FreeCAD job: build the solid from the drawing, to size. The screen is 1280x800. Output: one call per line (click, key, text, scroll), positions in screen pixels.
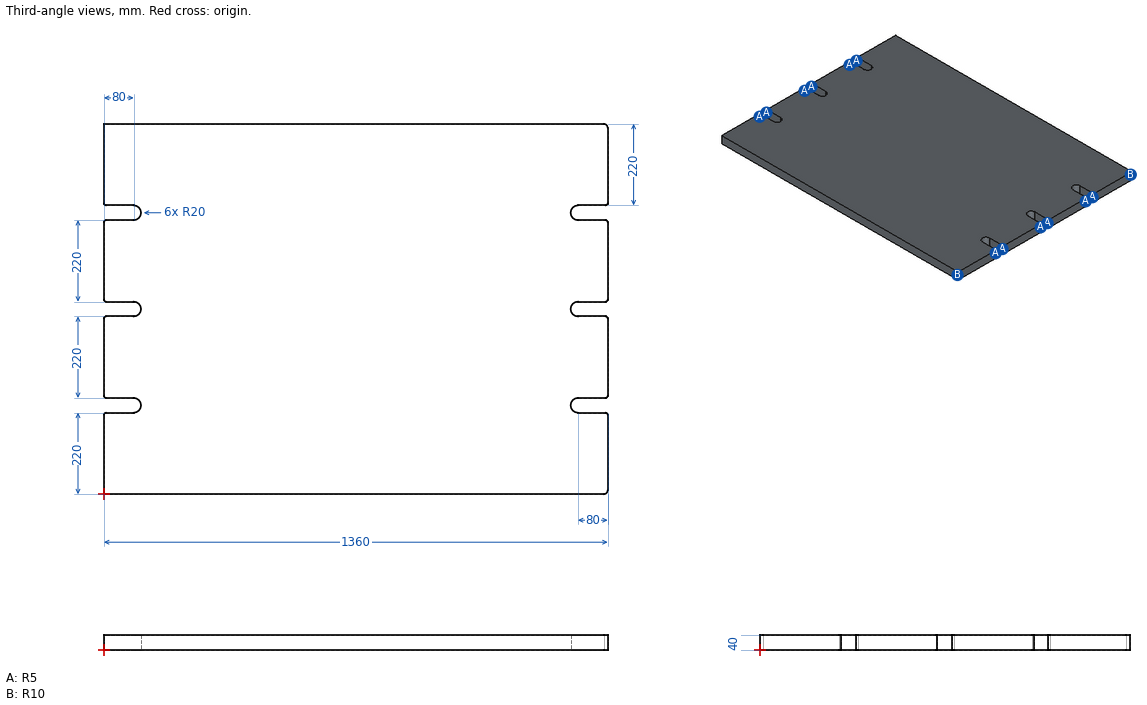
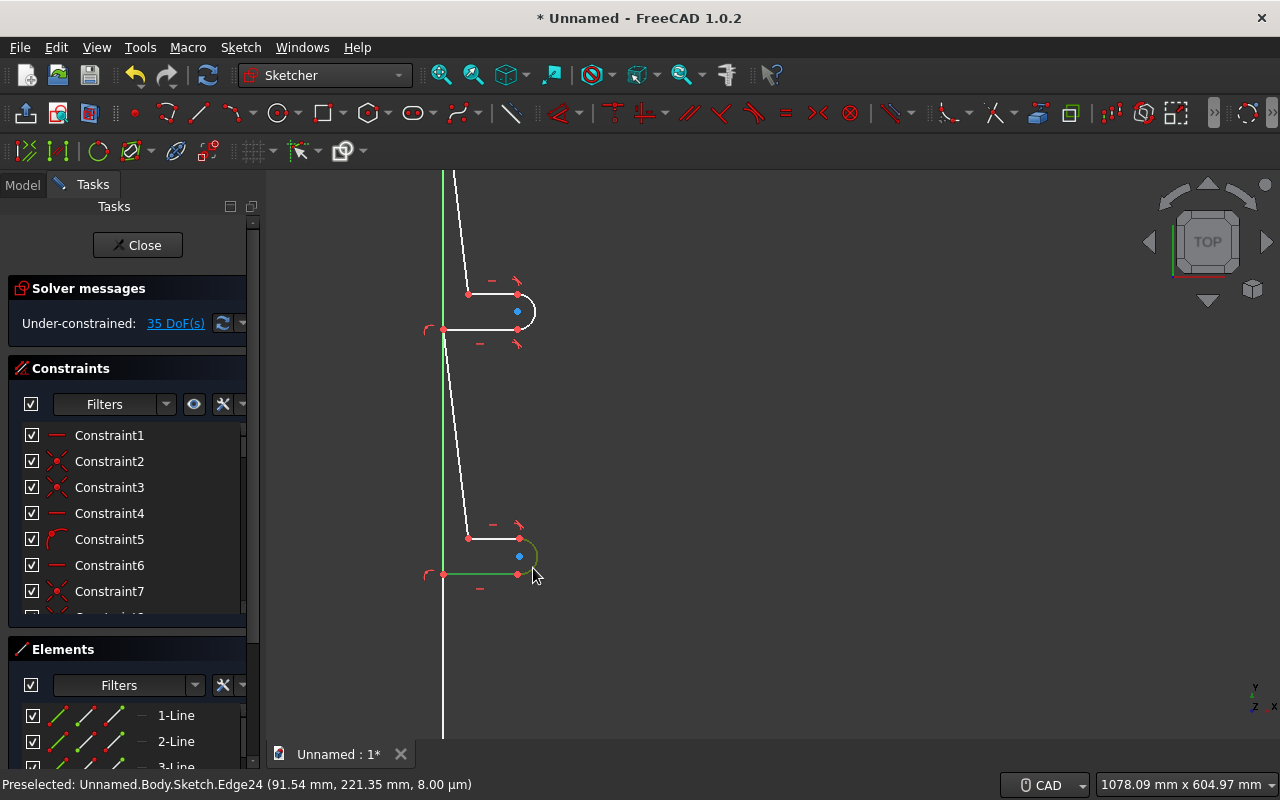
click(754, 114)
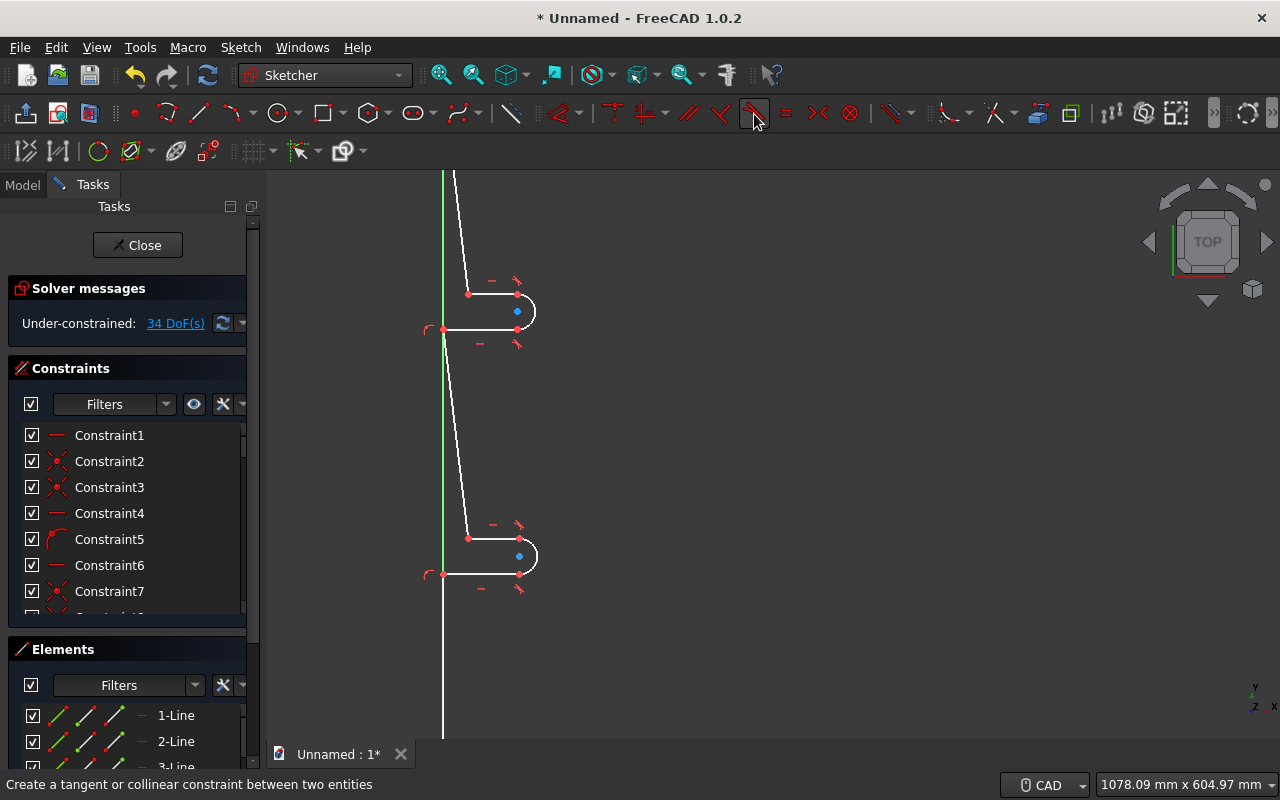
scroll(484, 539, down, 5)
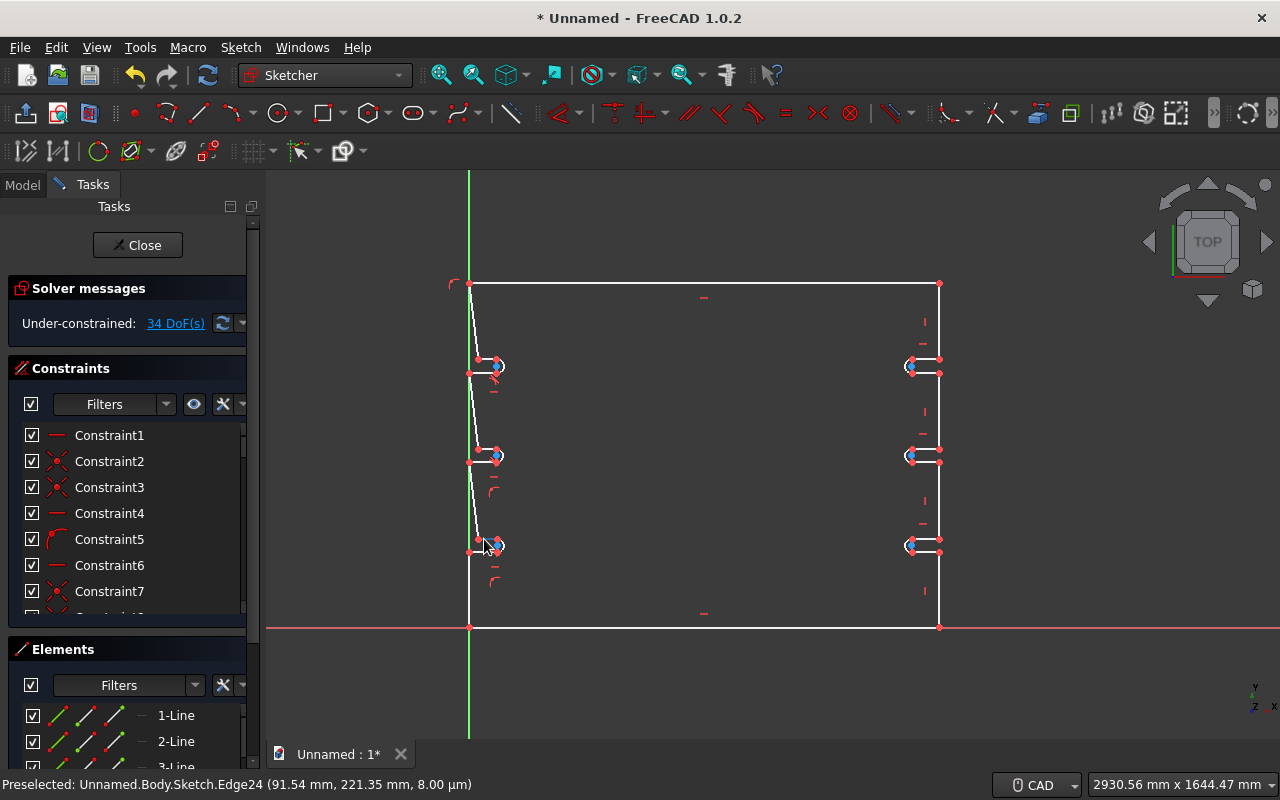
scroll(931, 552, up, 3)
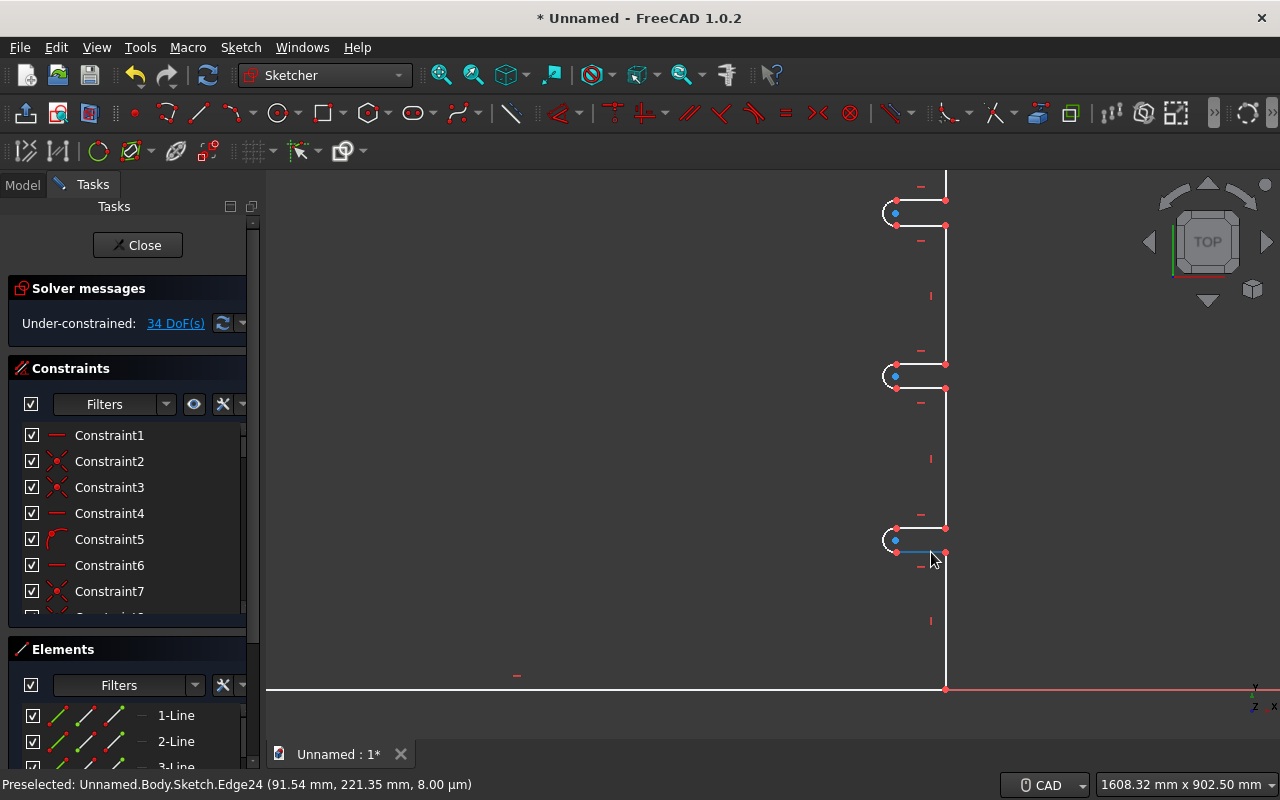
click(931, 552)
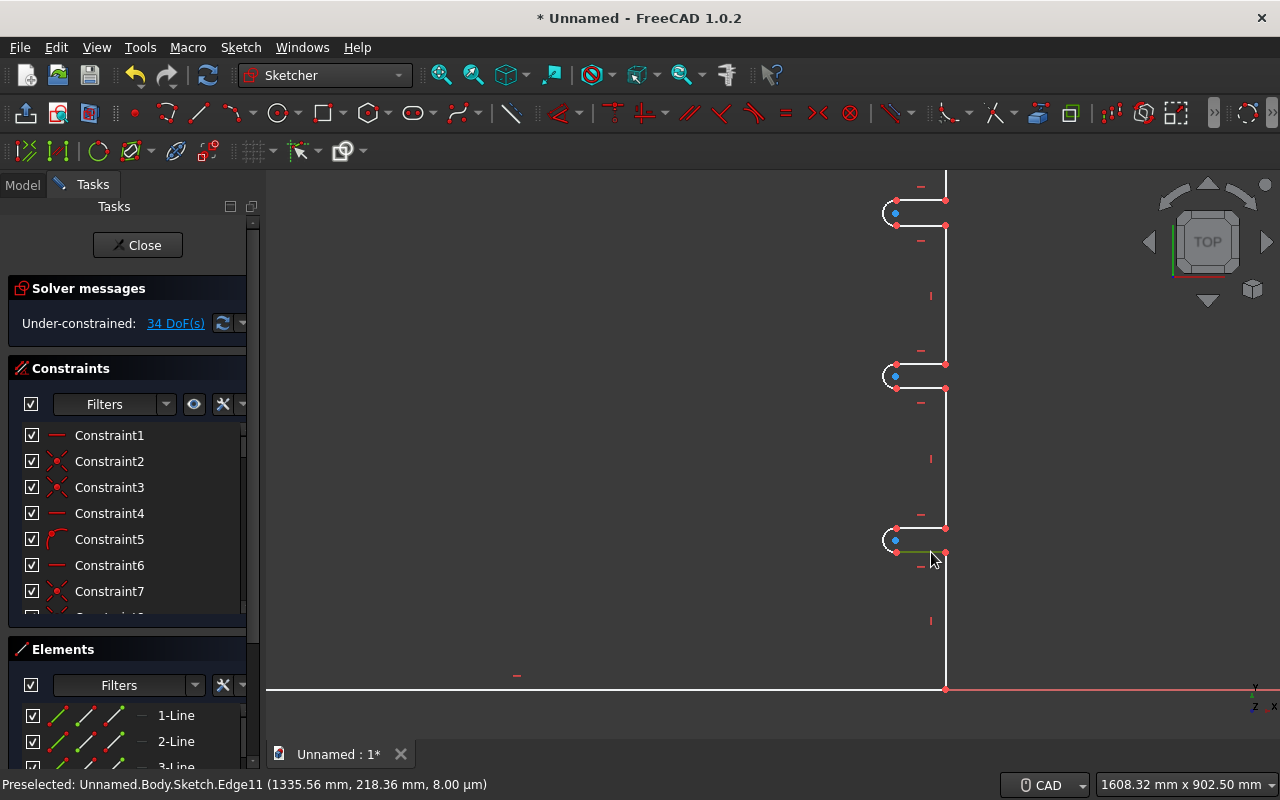
click(886, 533)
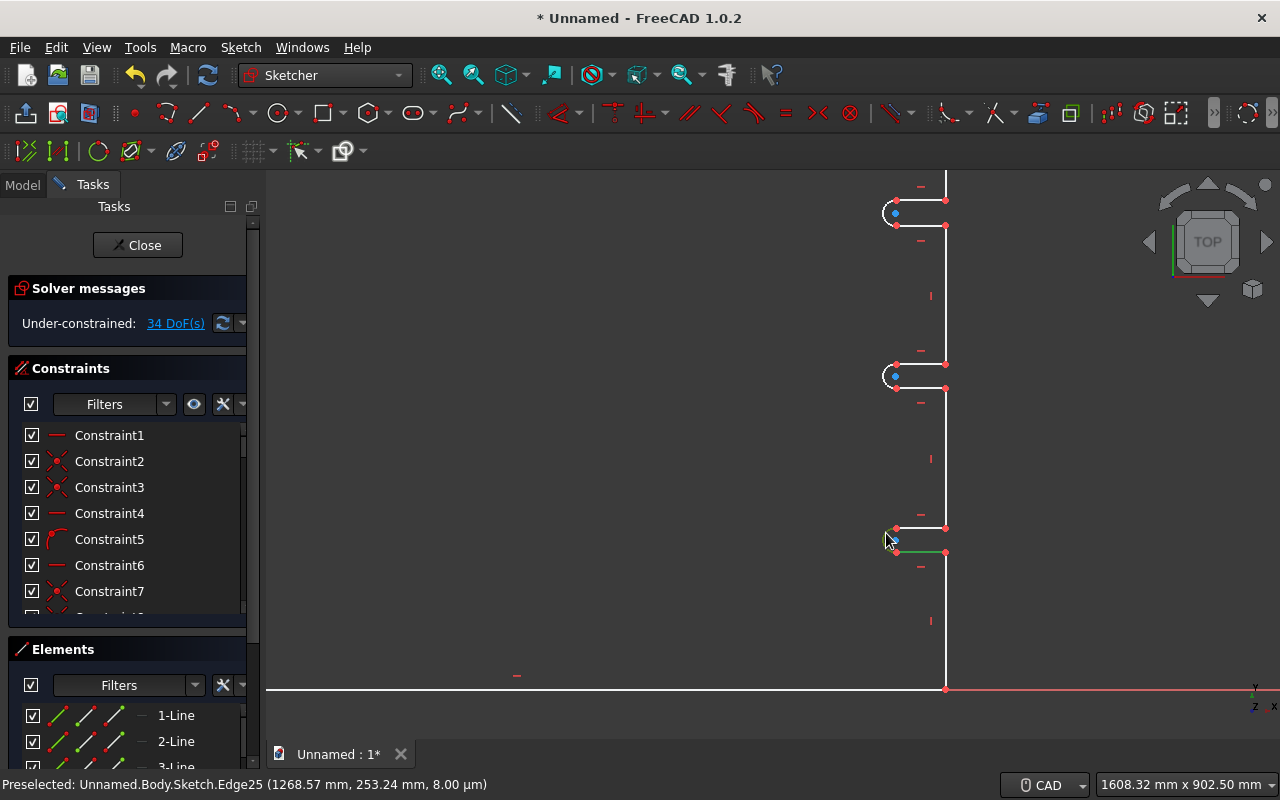
click(754, 114)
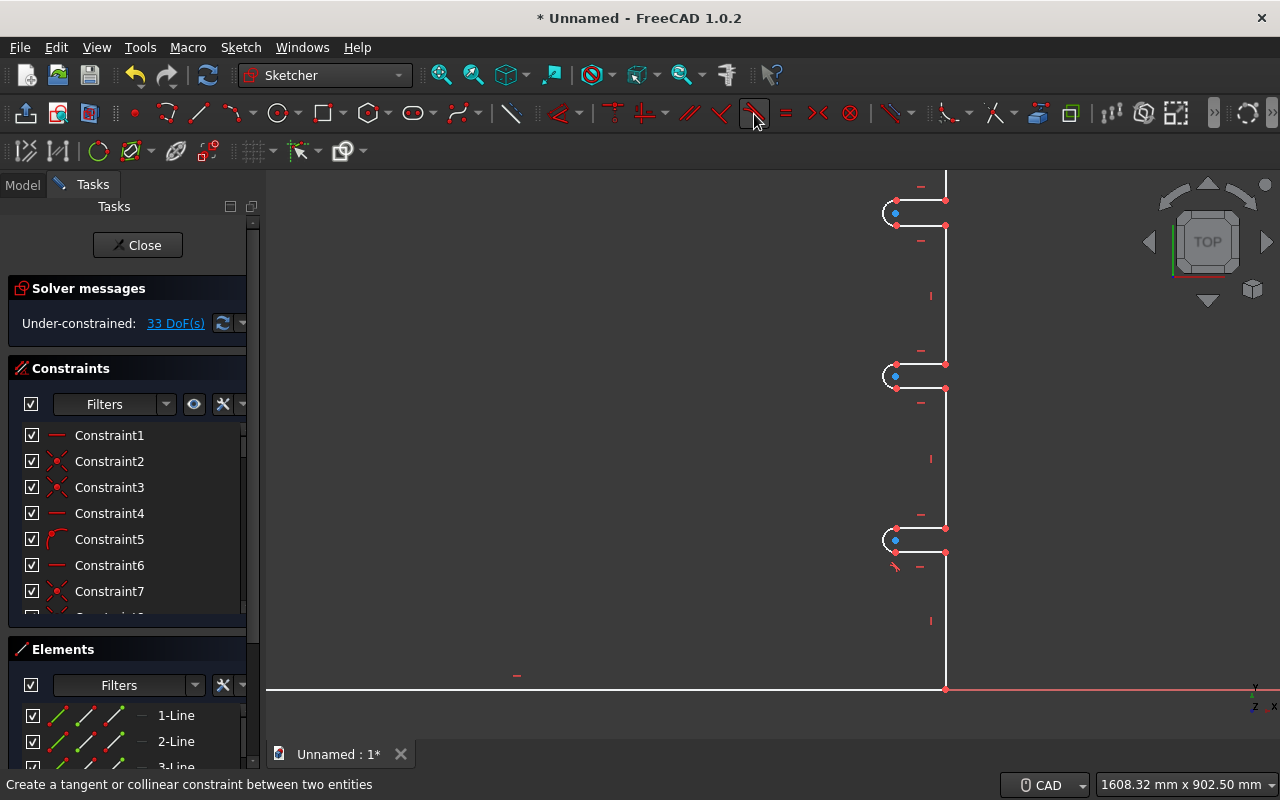
click(911, 528)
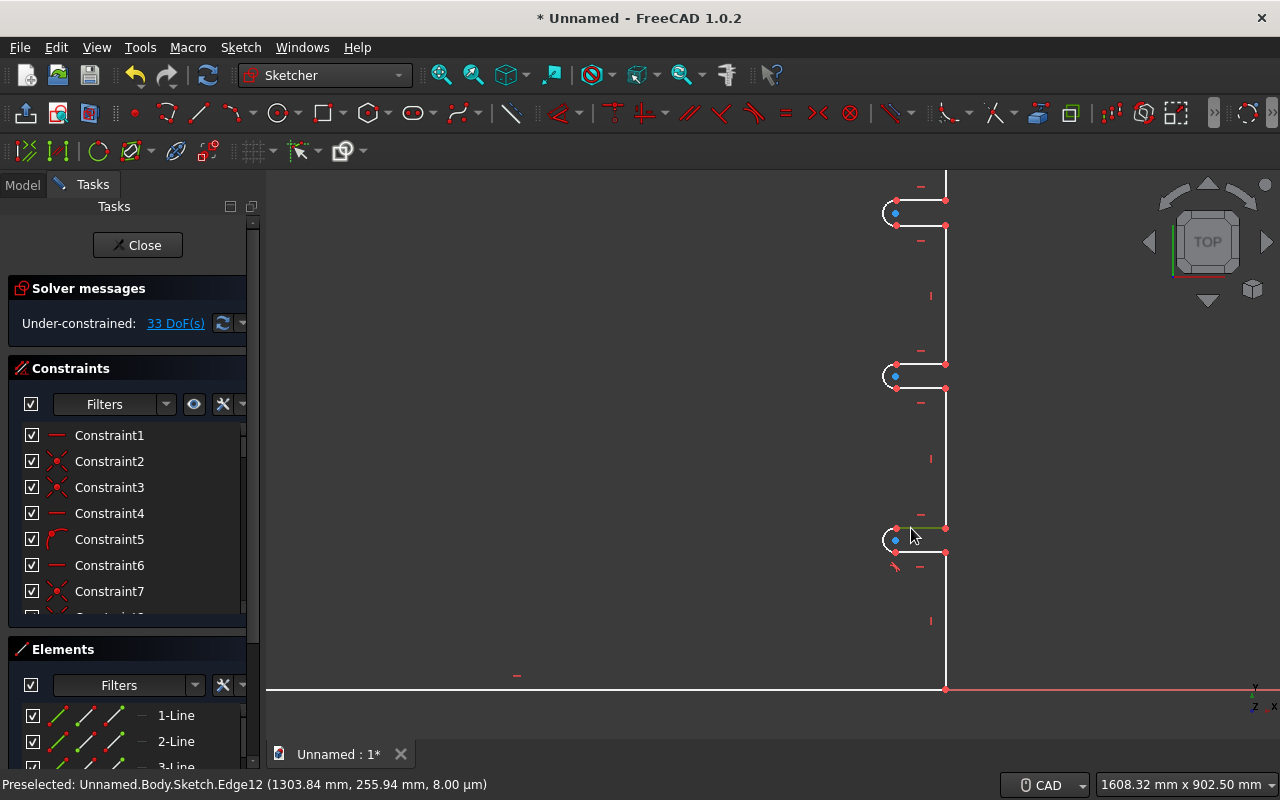
scroll(886, 532, up, 2)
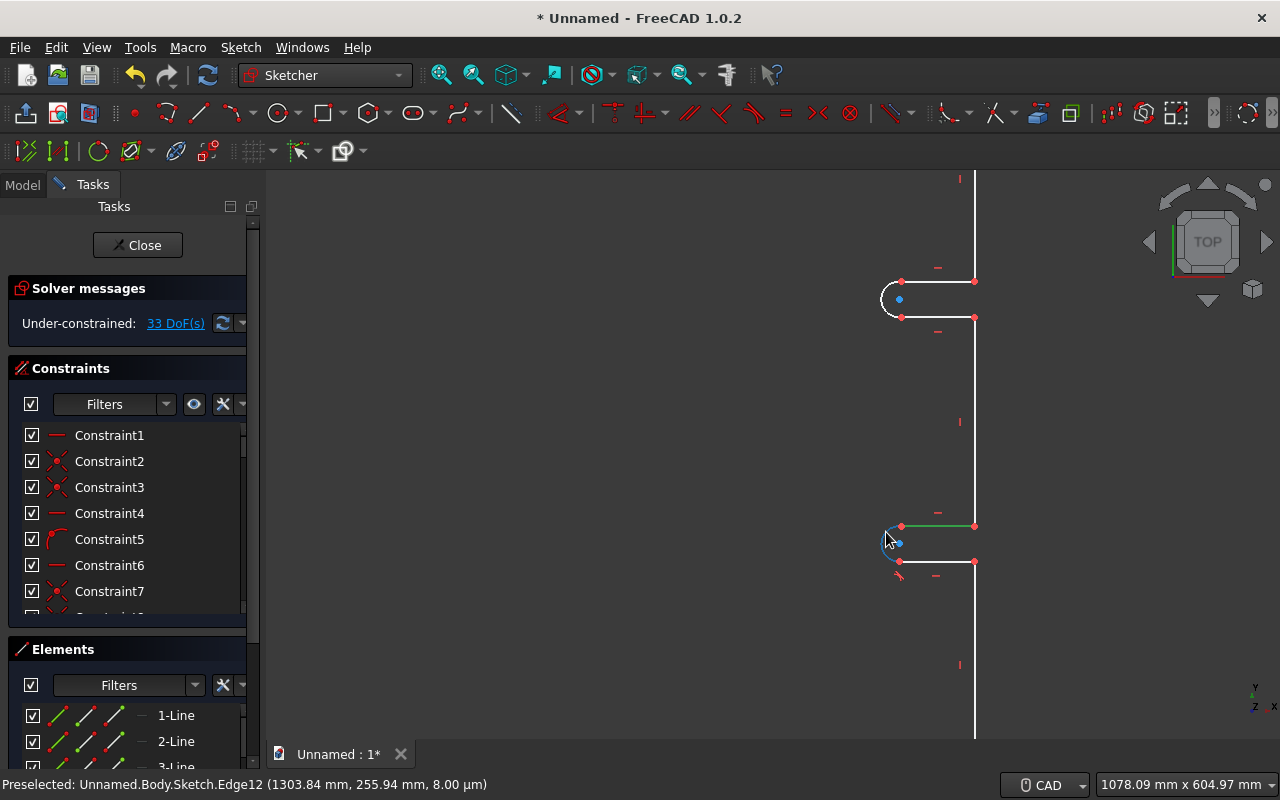
click(886, 532)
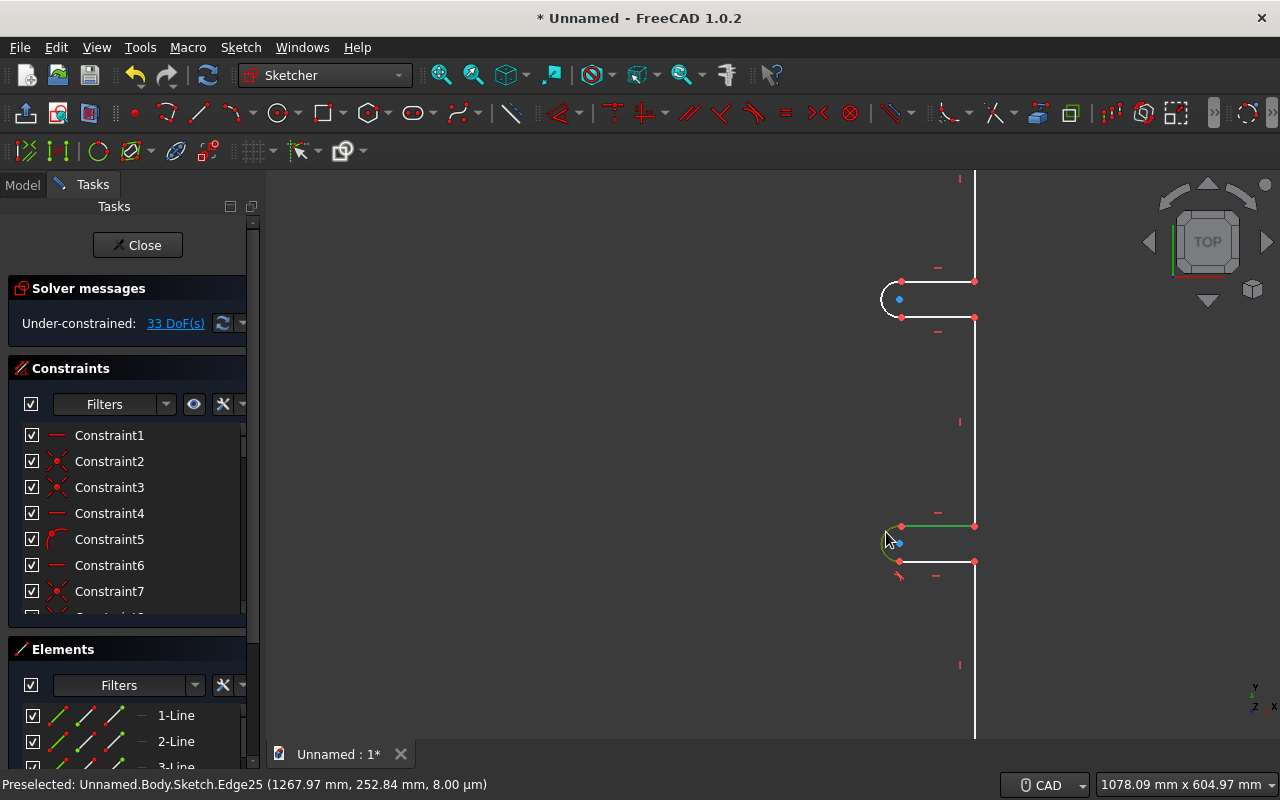
click(754, 114)